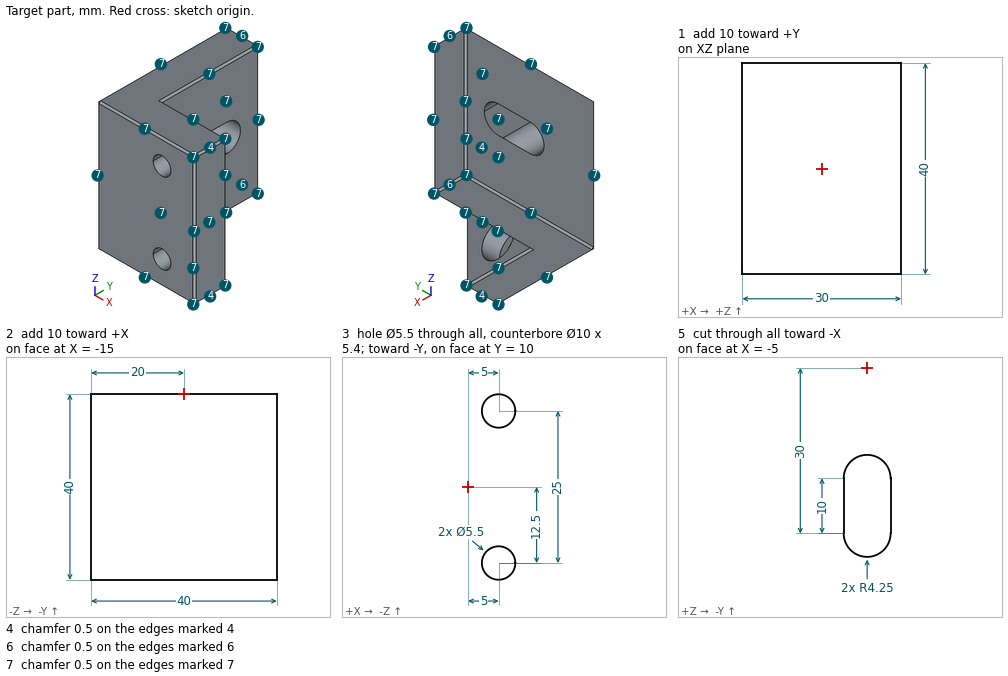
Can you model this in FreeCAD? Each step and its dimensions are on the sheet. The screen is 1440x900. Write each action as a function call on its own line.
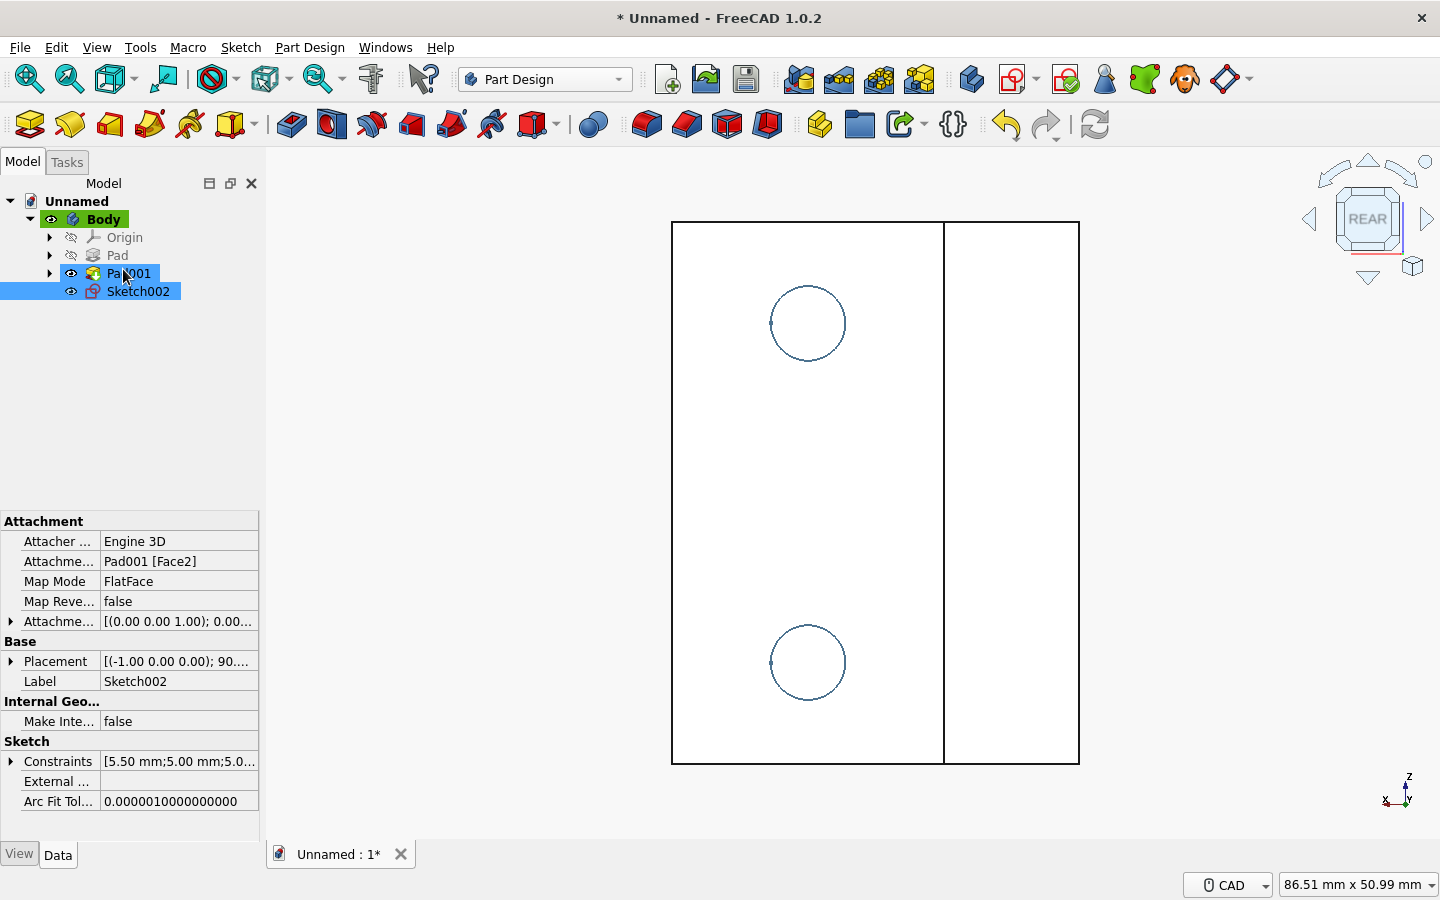
click(332, 124)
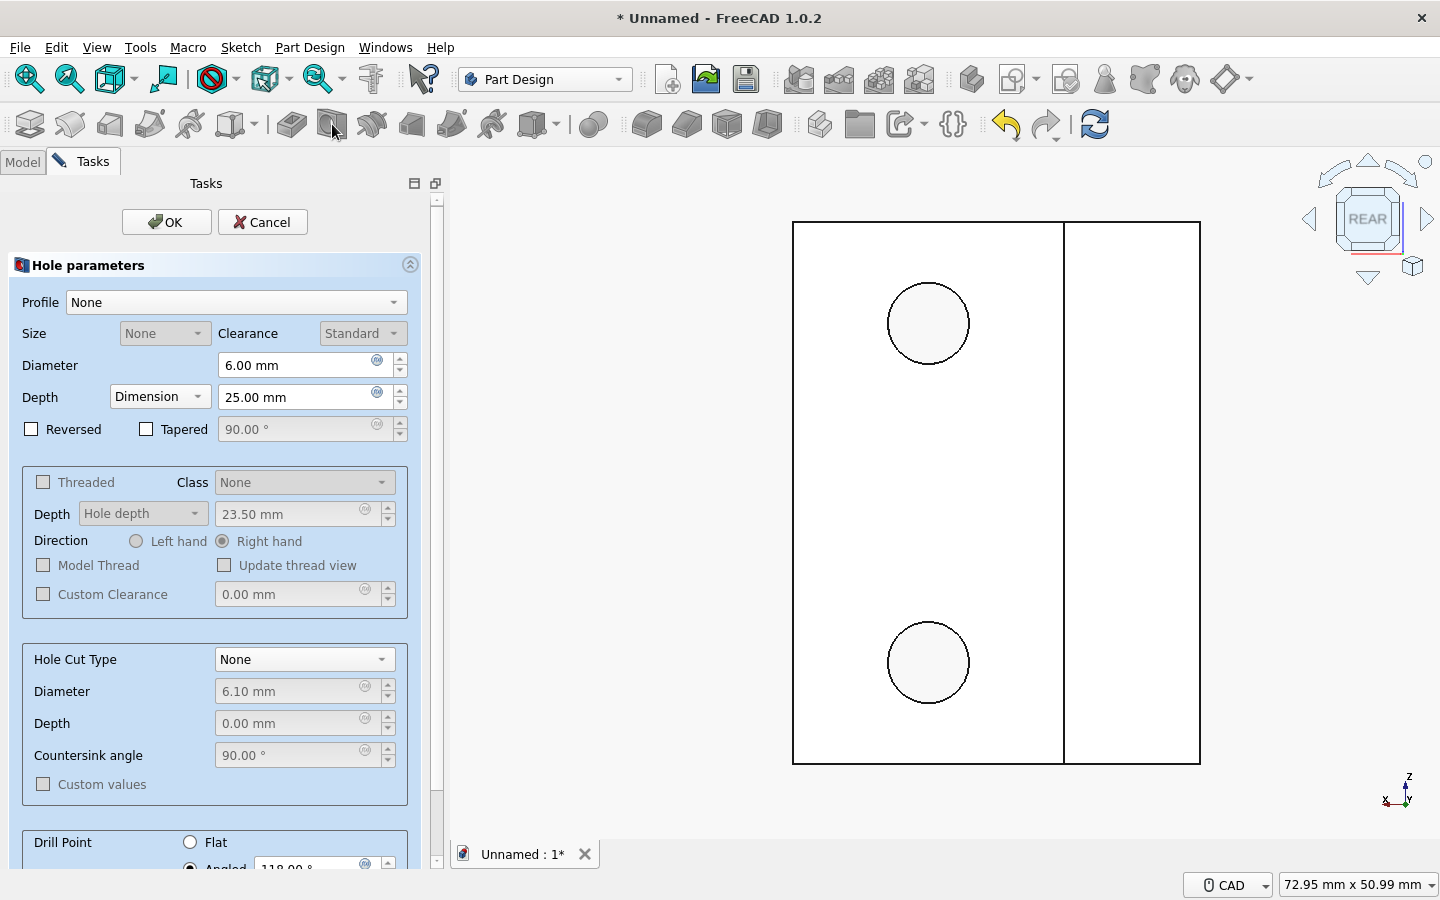
triple_click(305, 365)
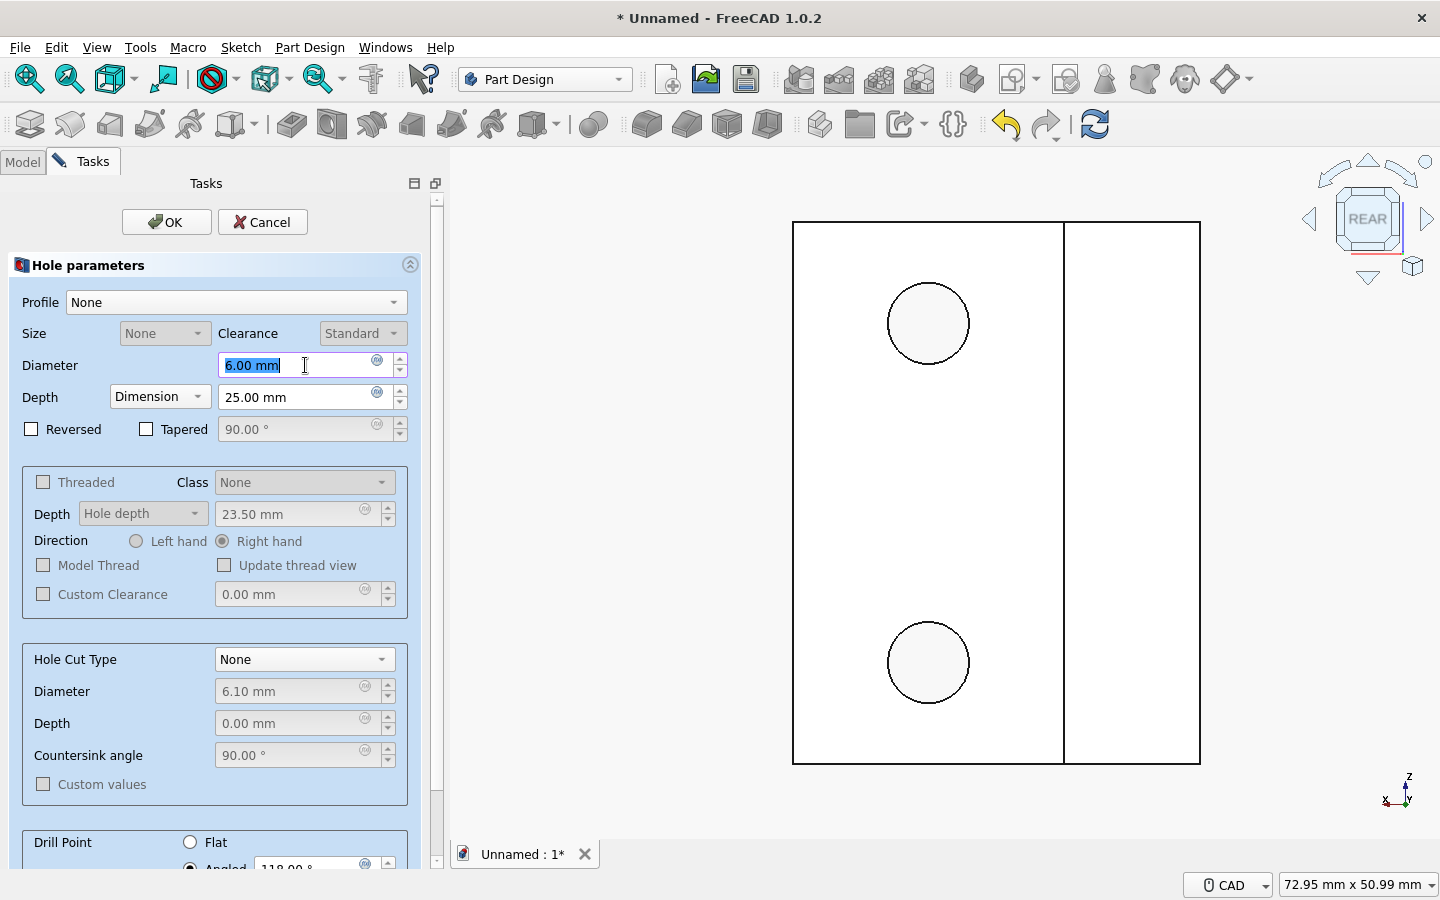
text(5.5)
key(Tab)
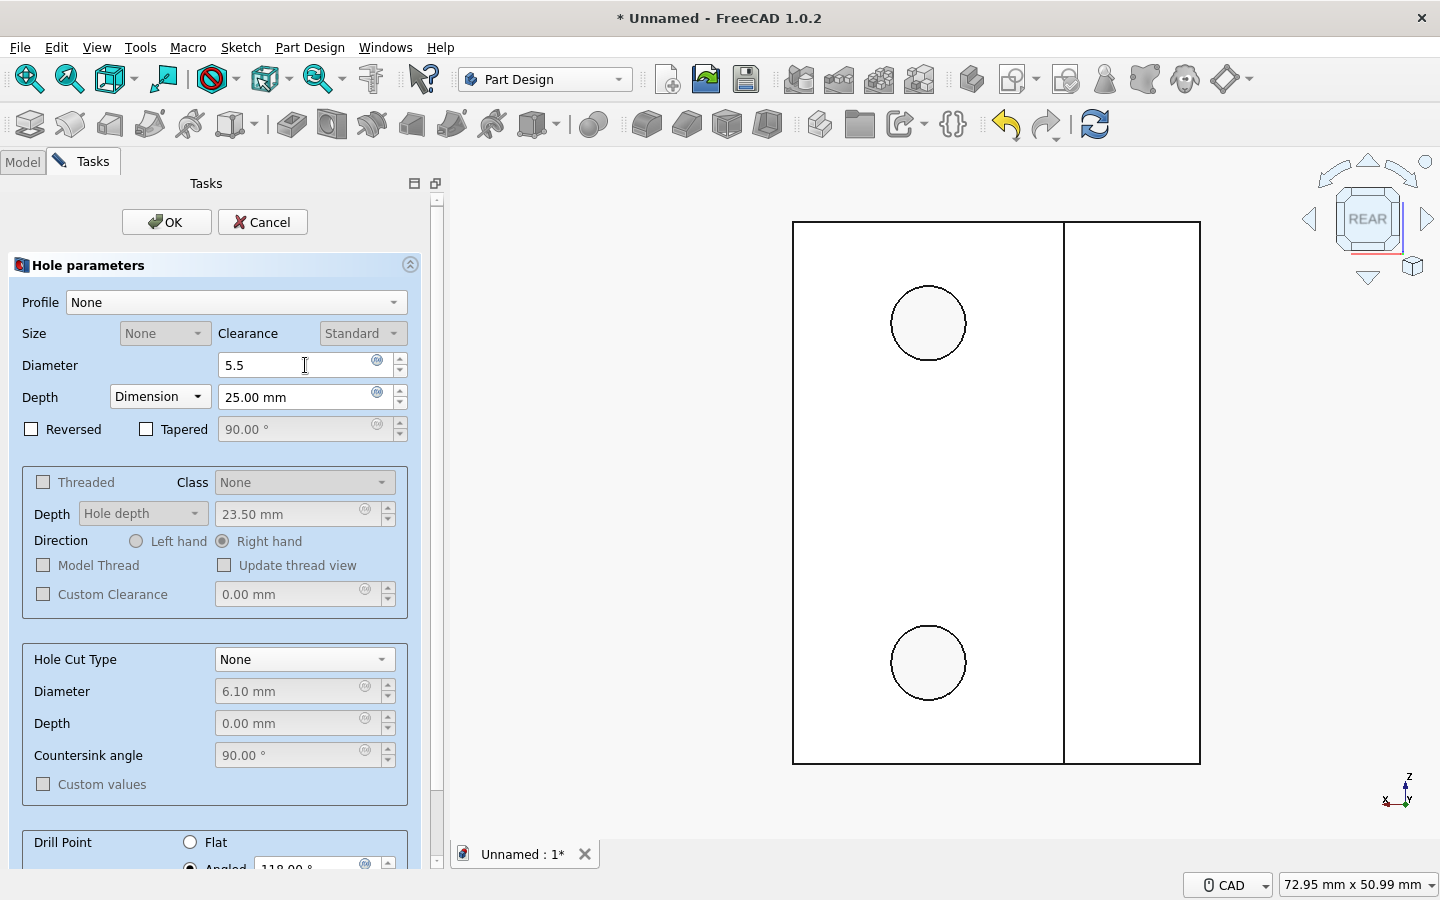
click(161, 396)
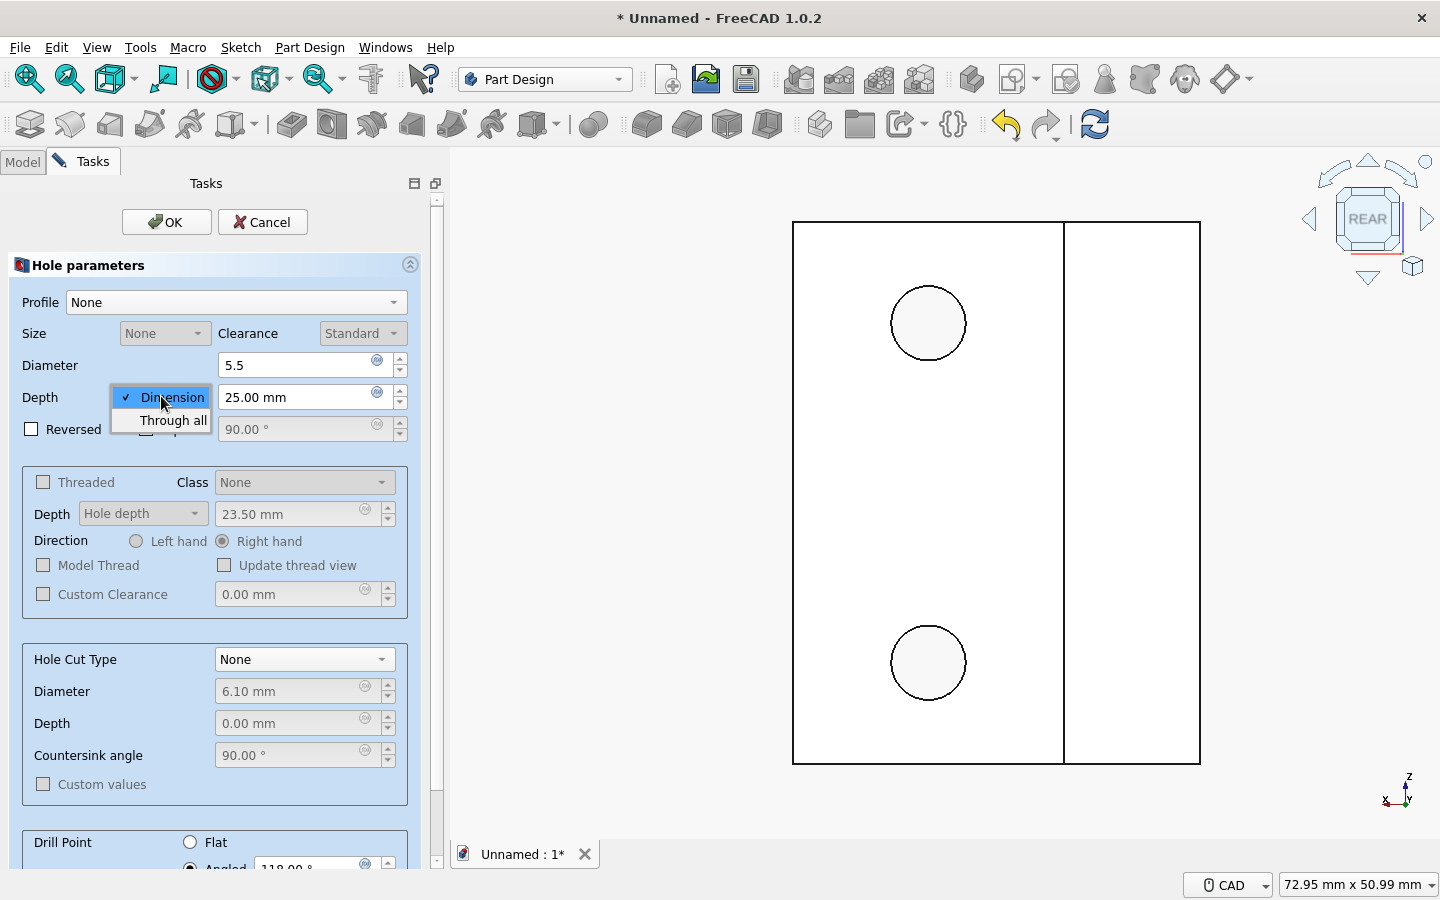
click(160, 420)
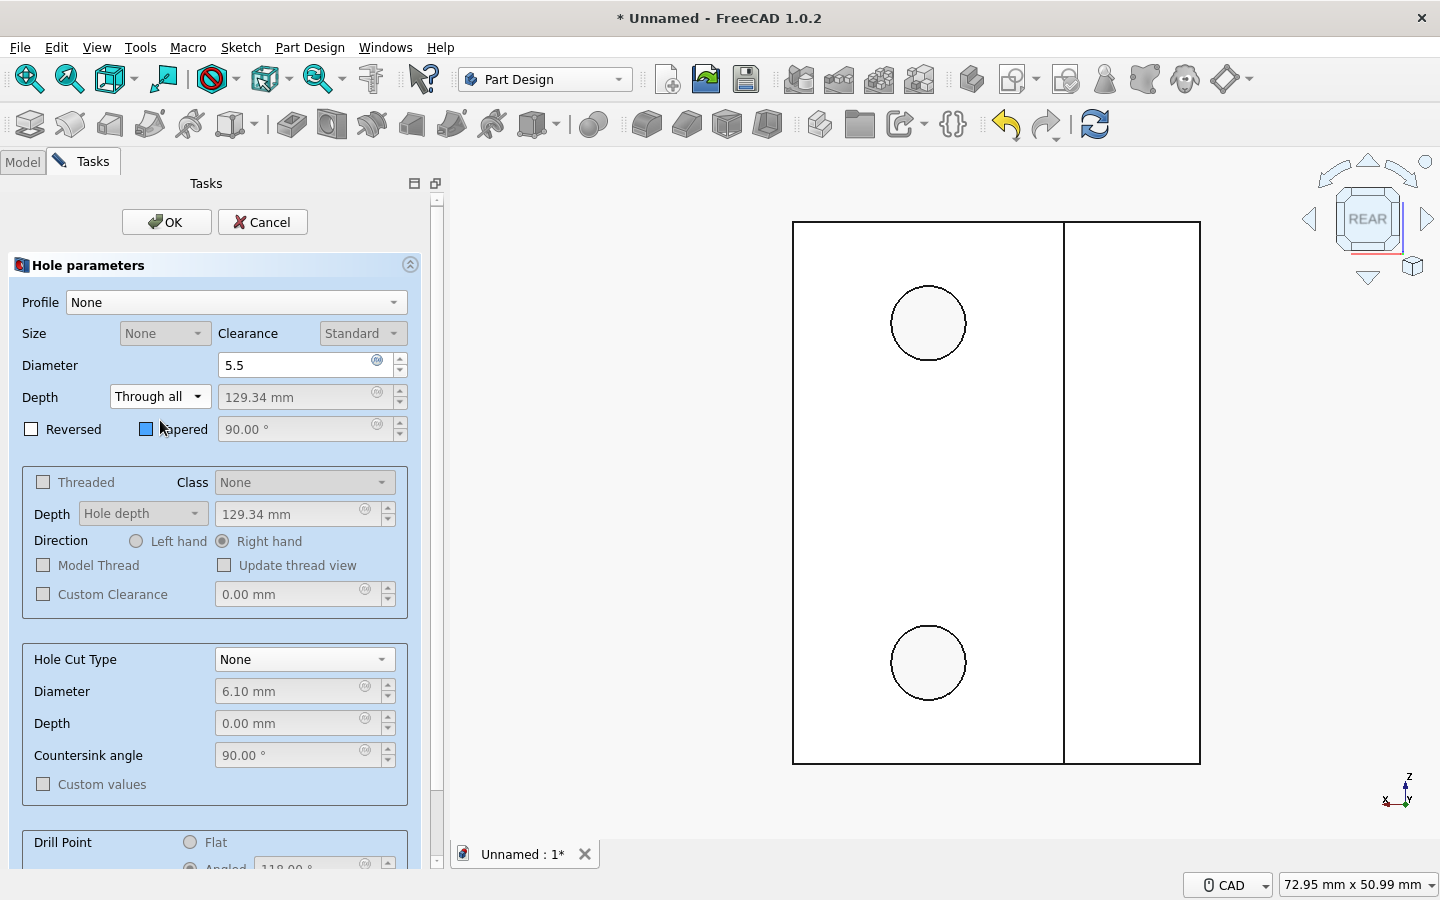
click(306, 660)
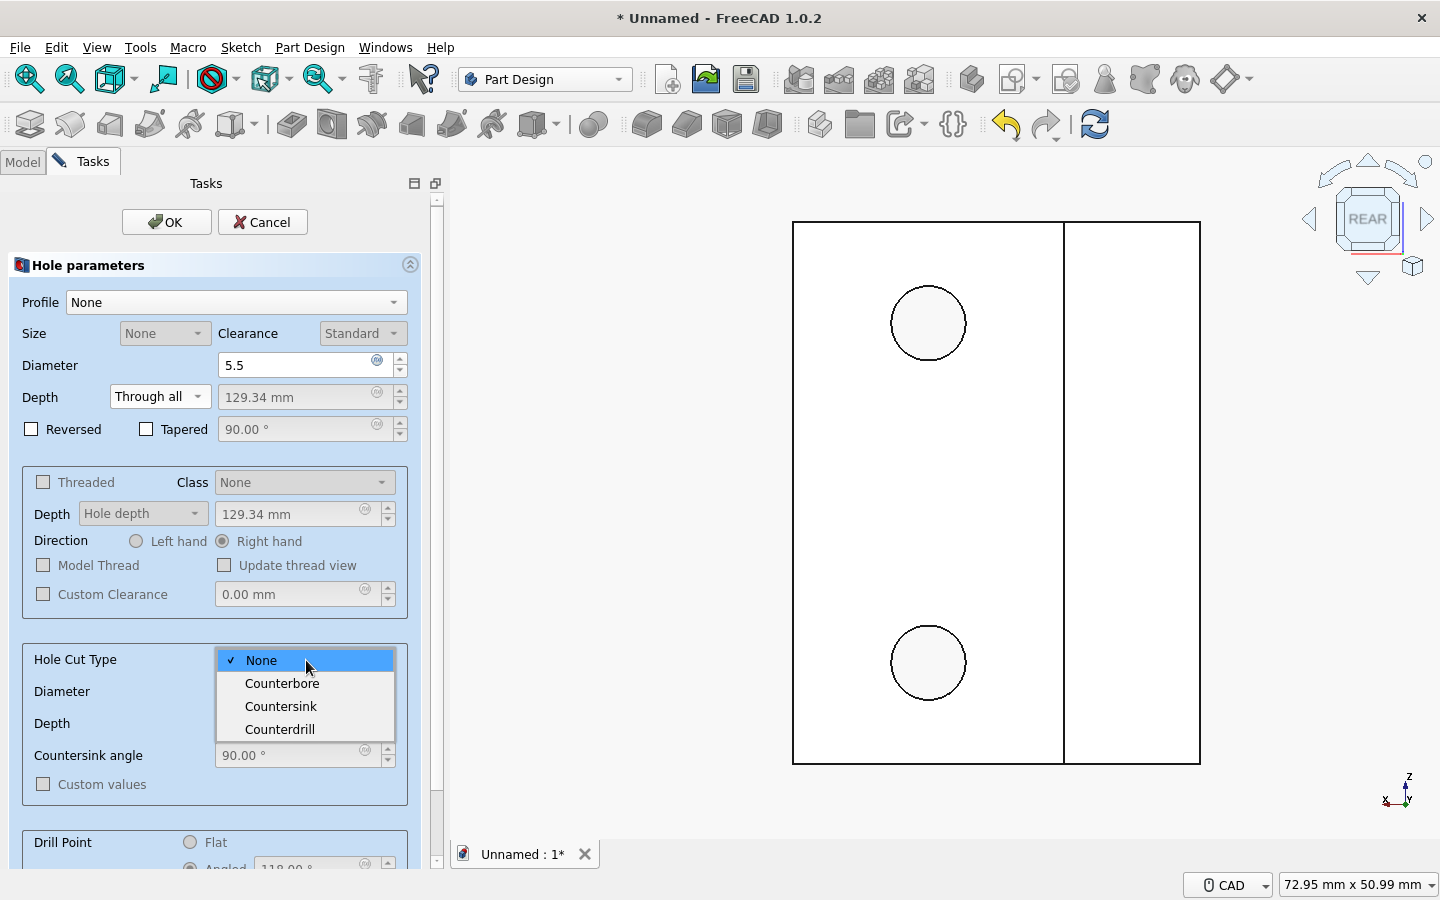
click(304, 684)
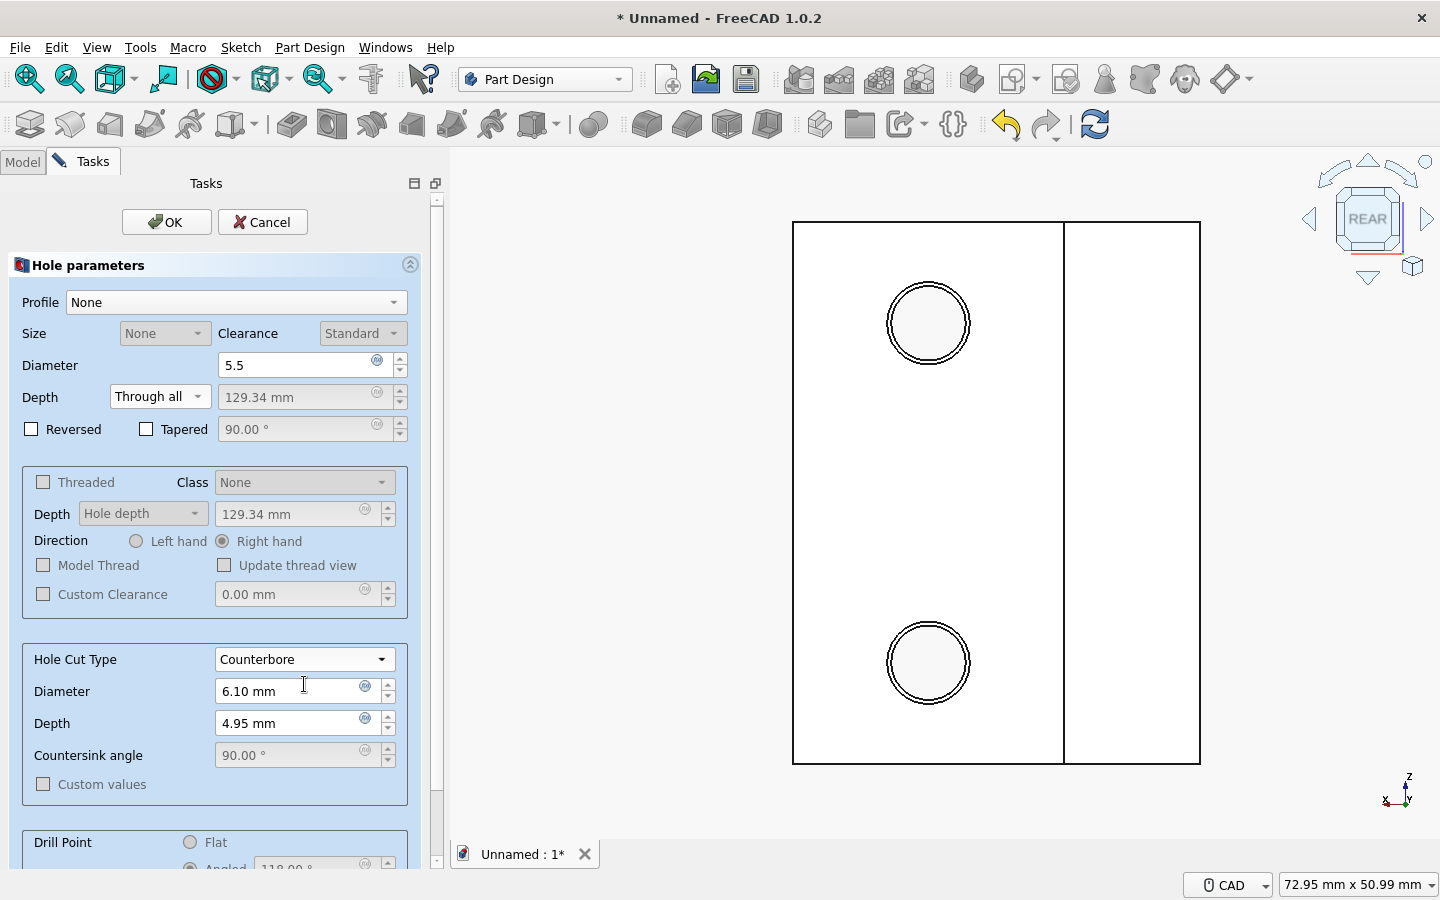
triple_click(298, 691)